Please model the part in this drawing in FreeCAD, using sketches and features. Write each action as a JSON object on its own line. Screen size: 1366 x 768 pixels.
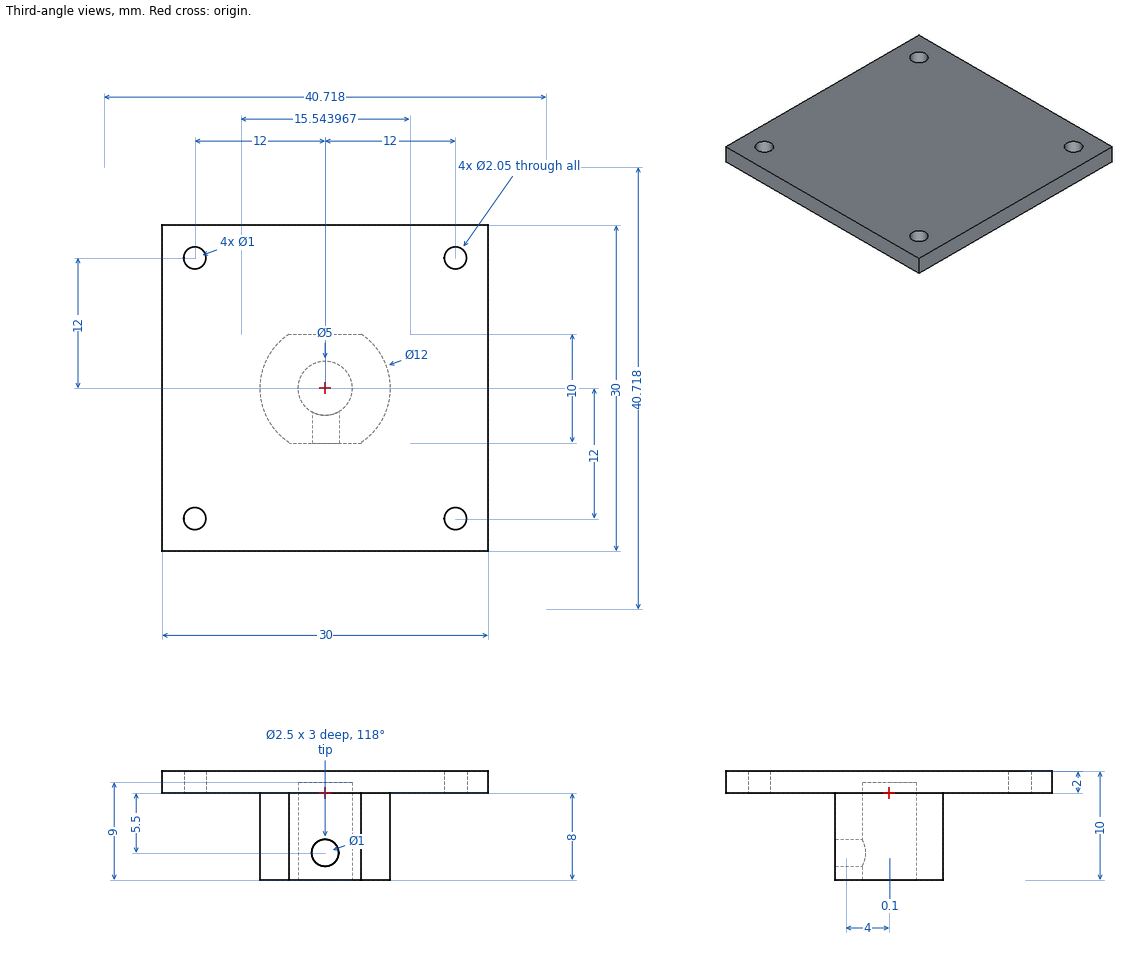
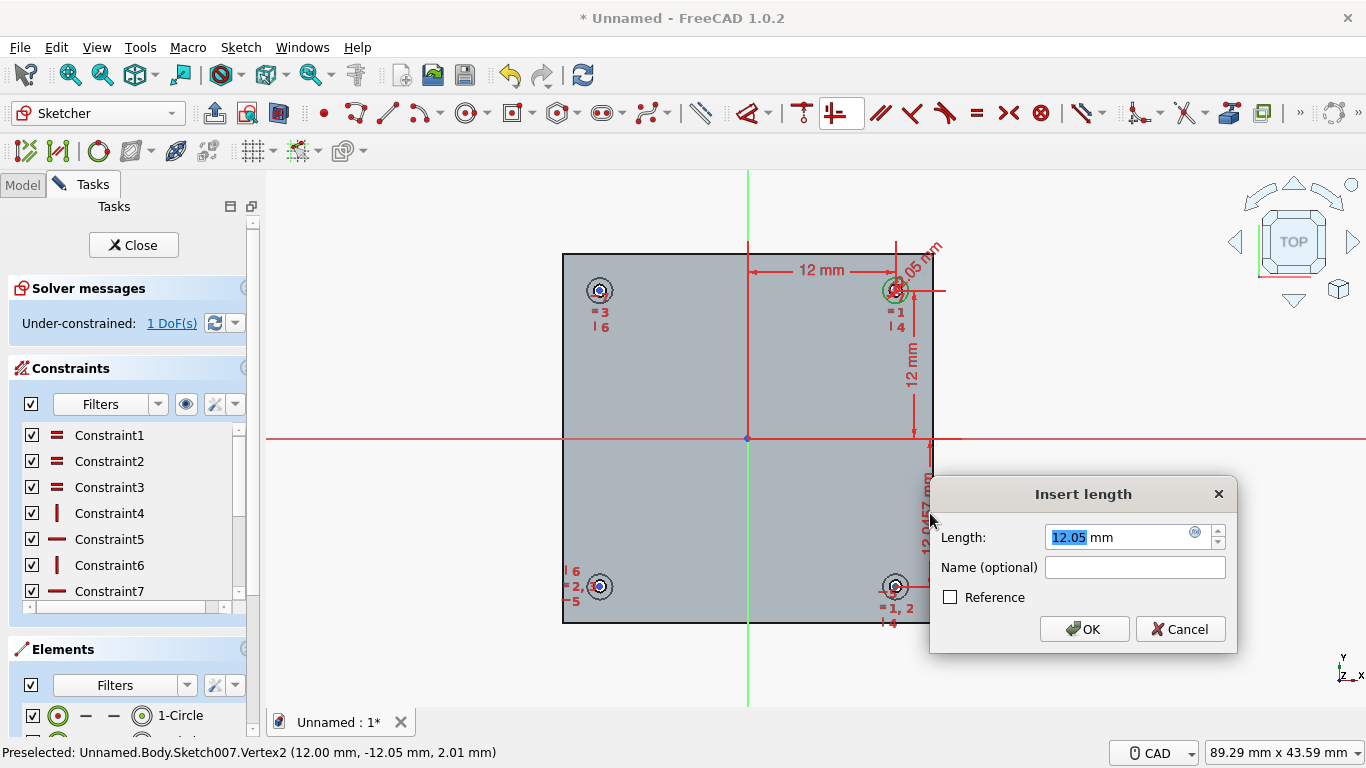
{"action": "type", "text": "12"}
{"action": "key", "text": "Return"}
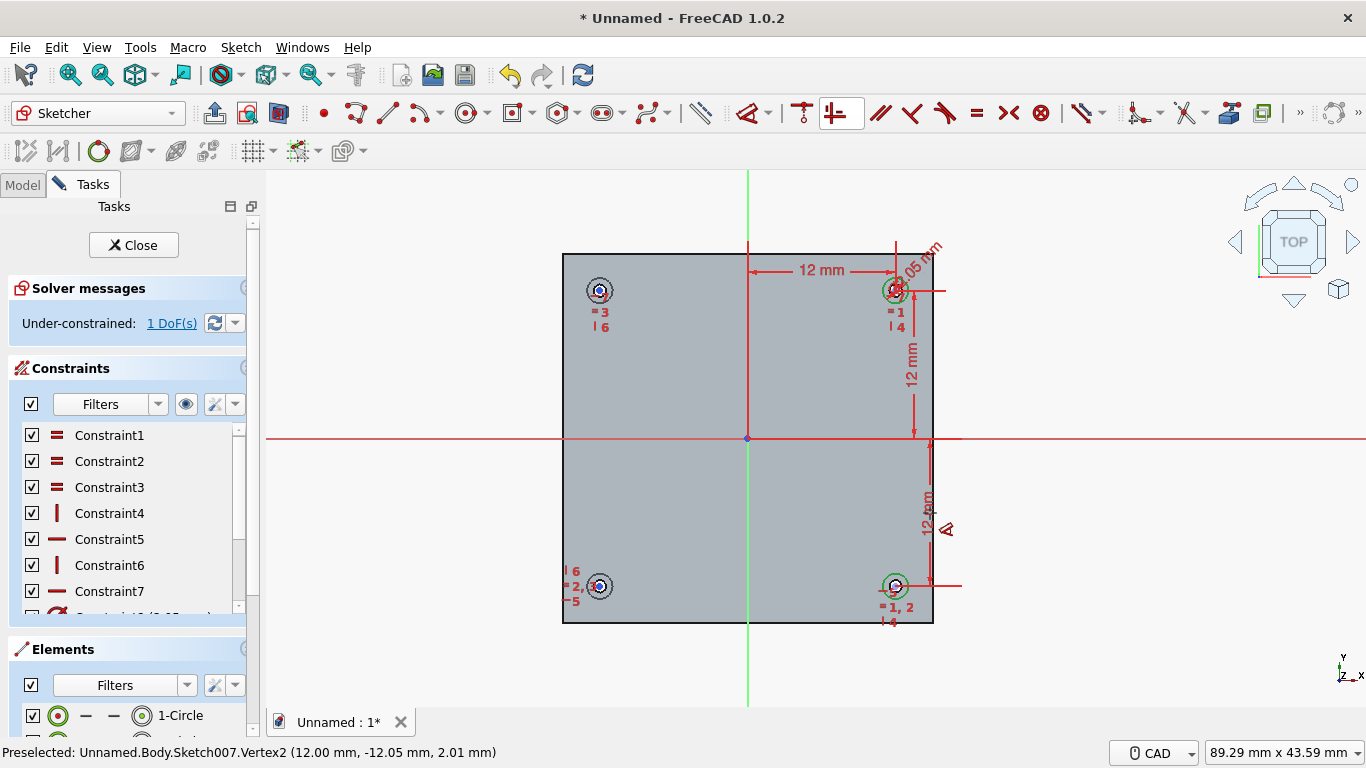
{"action": "left_click", "coordinate": [600, 586]}
{"action": "left_click", "coordinate": [674, 620]}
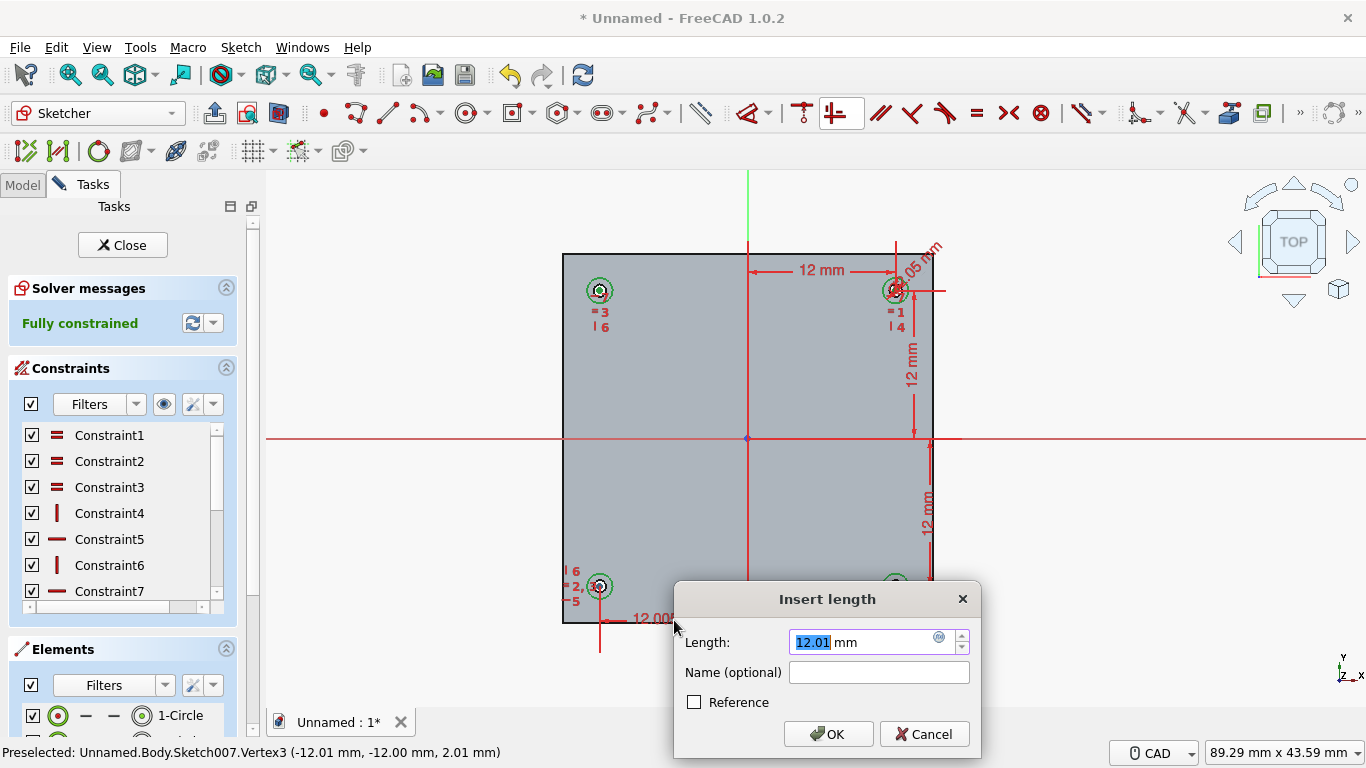
{"action": "type", "text": "12"}
{"action": "key", "text": "Return"}
{"action": "key", "text": "Escape"}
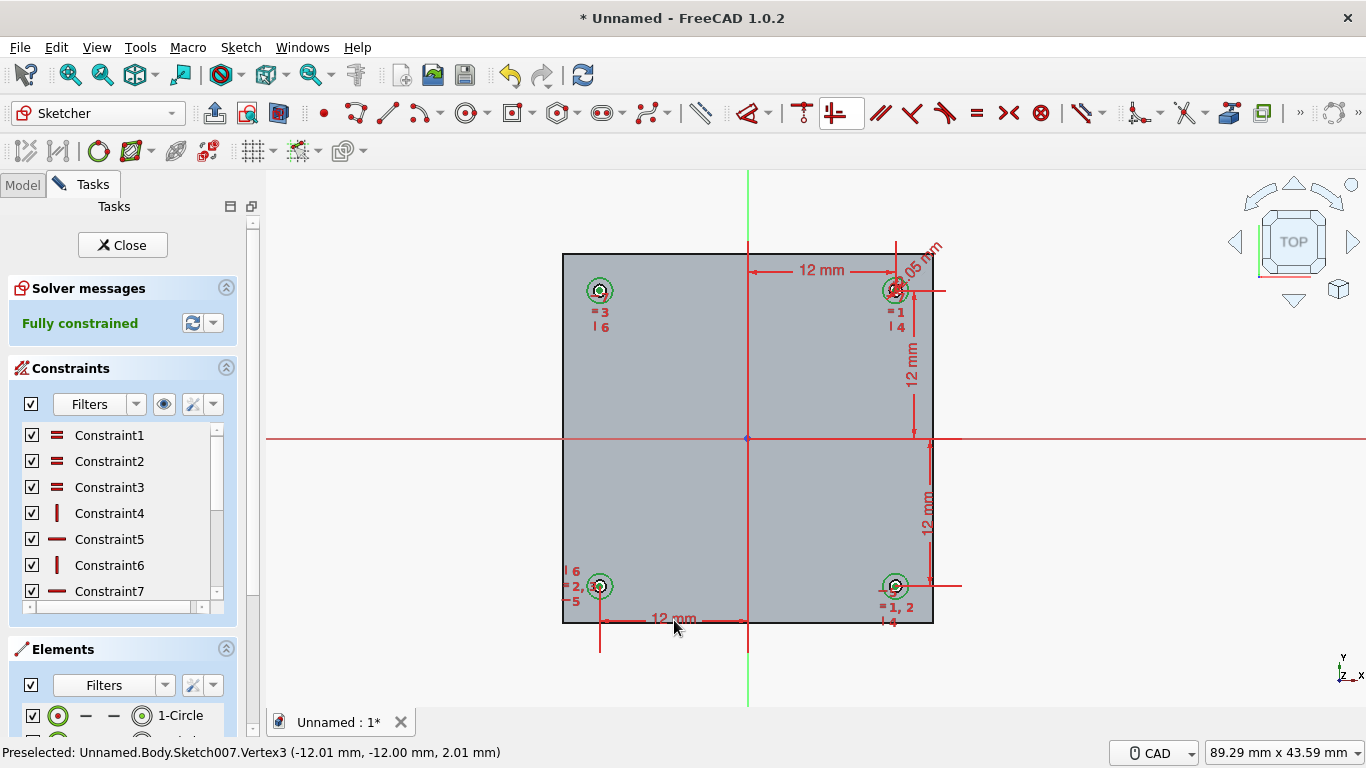
{"action": "left_click", "coordinate": [123, 245]}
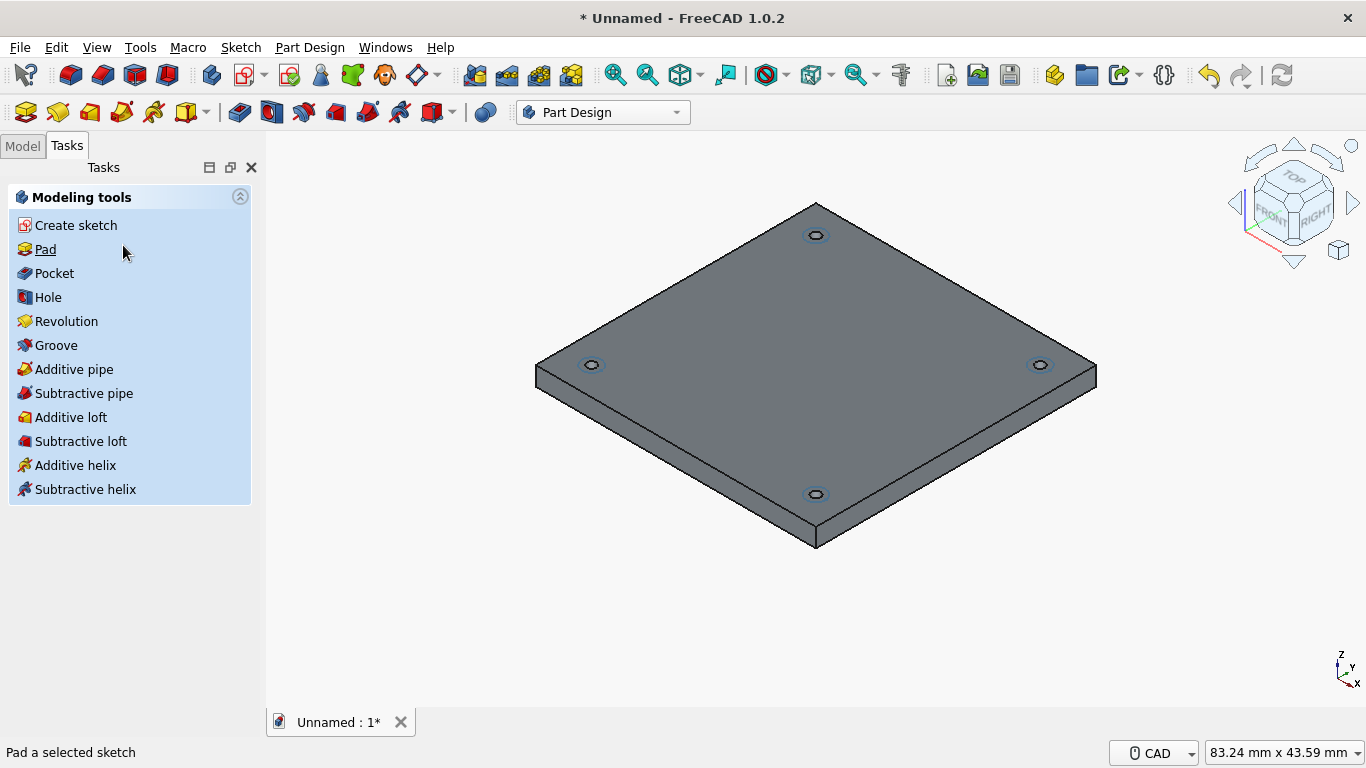
{"action": "left_click", "coordinate": [272, 112]}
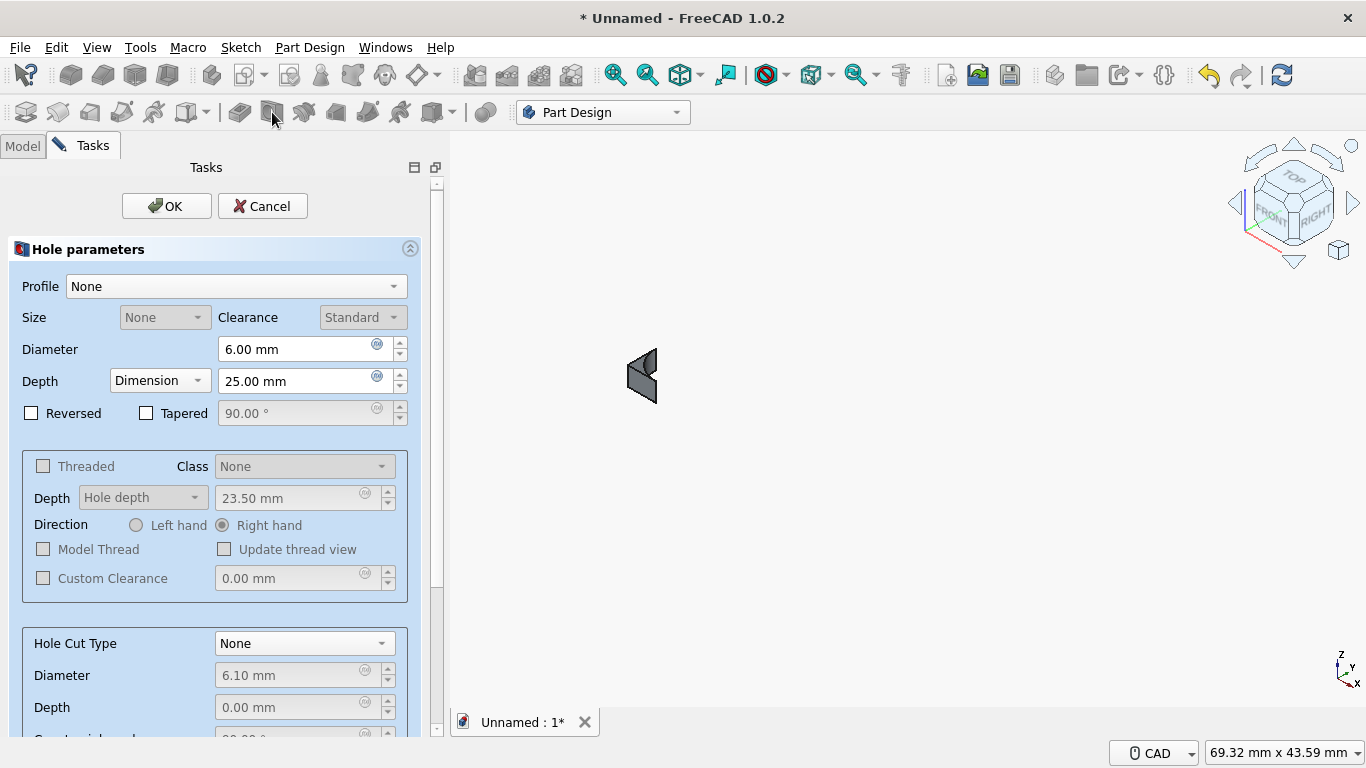
{"action": "triple_click", "coordinate": [305, 349]}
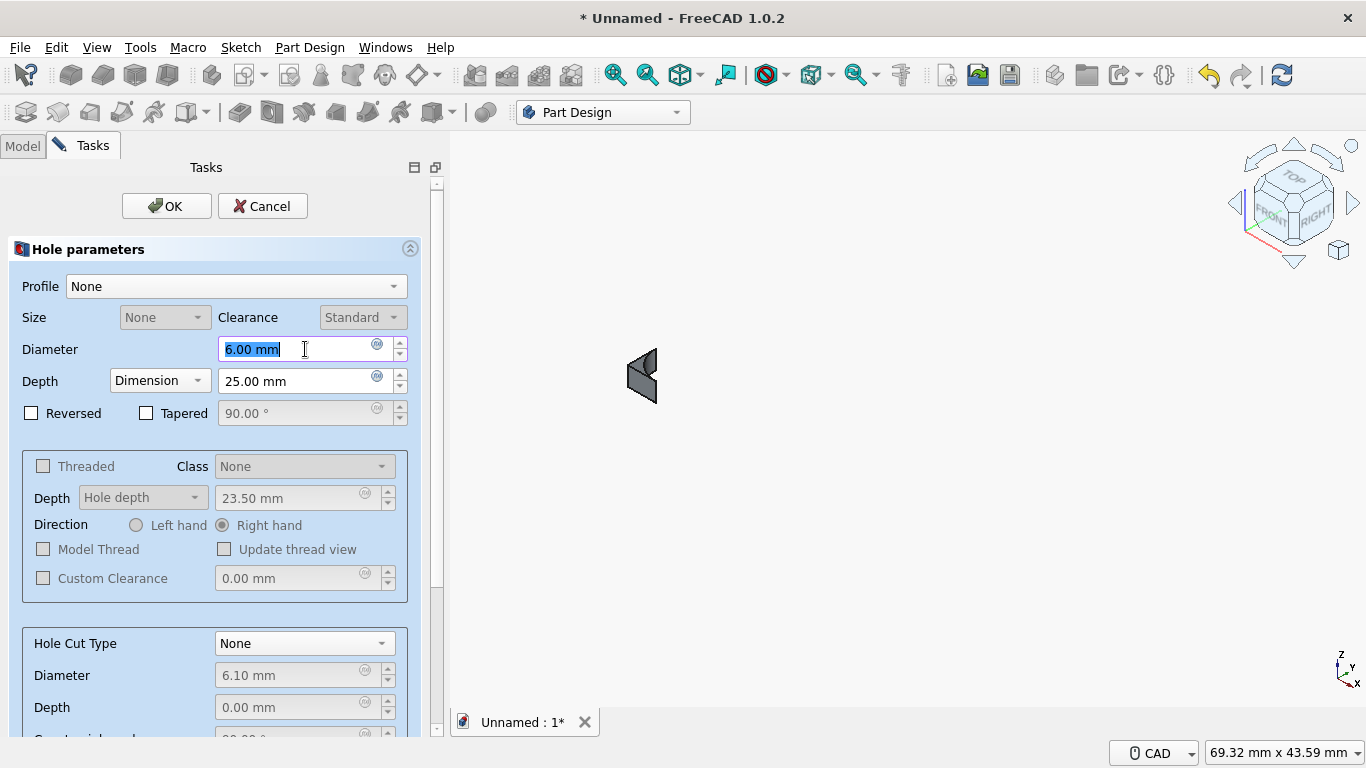
{"action": "type", "text": "2.05"}
{"action": "key", "text": "Tab"}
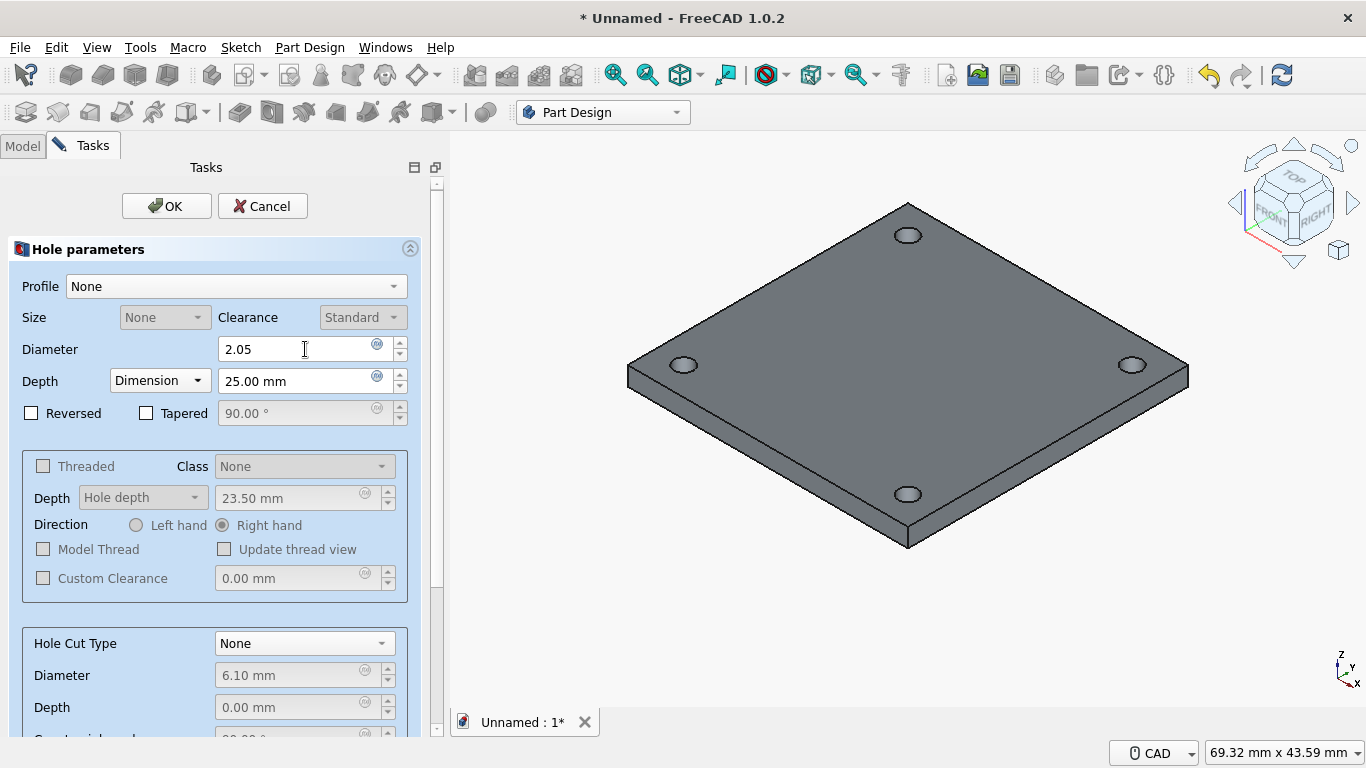
{"action": "left_click", "coordinate": [161, 380]}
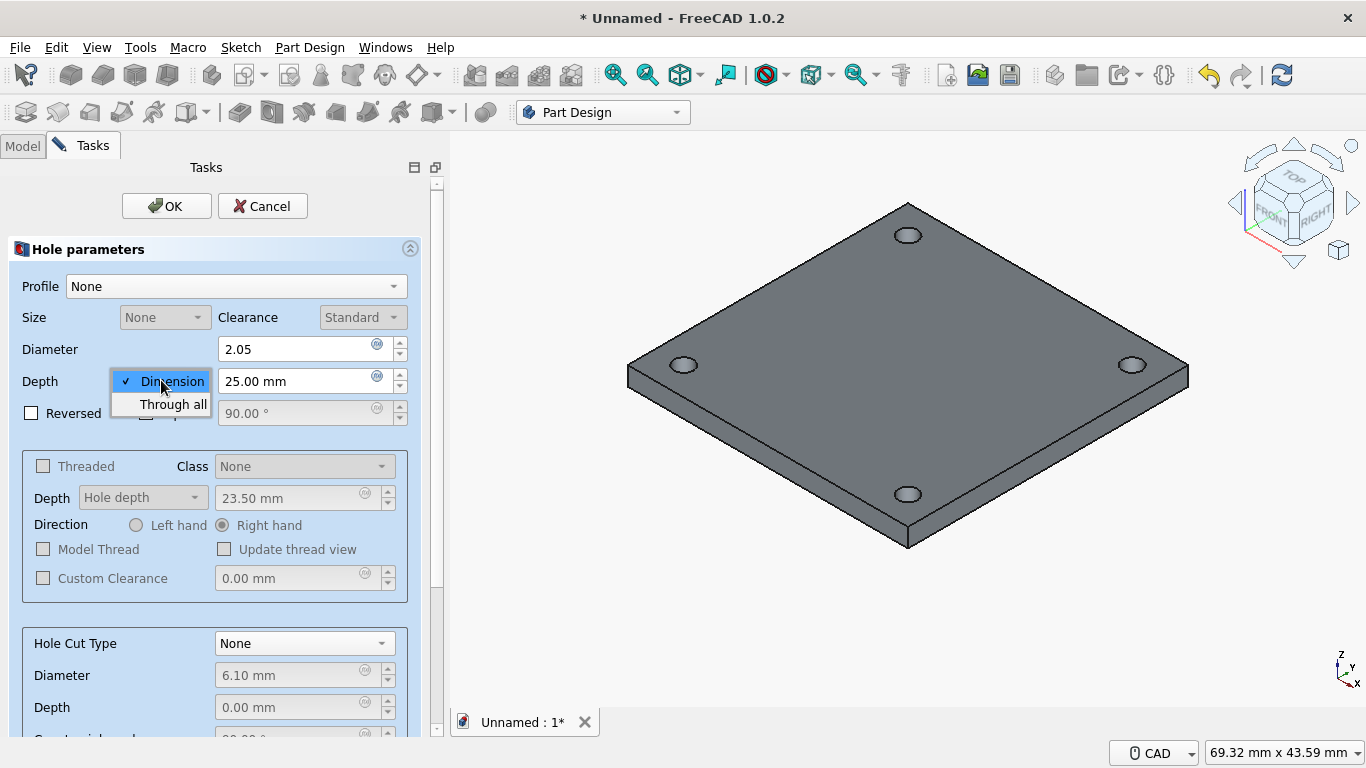
{"action": "left_click", "coordinate": [160, 404]}